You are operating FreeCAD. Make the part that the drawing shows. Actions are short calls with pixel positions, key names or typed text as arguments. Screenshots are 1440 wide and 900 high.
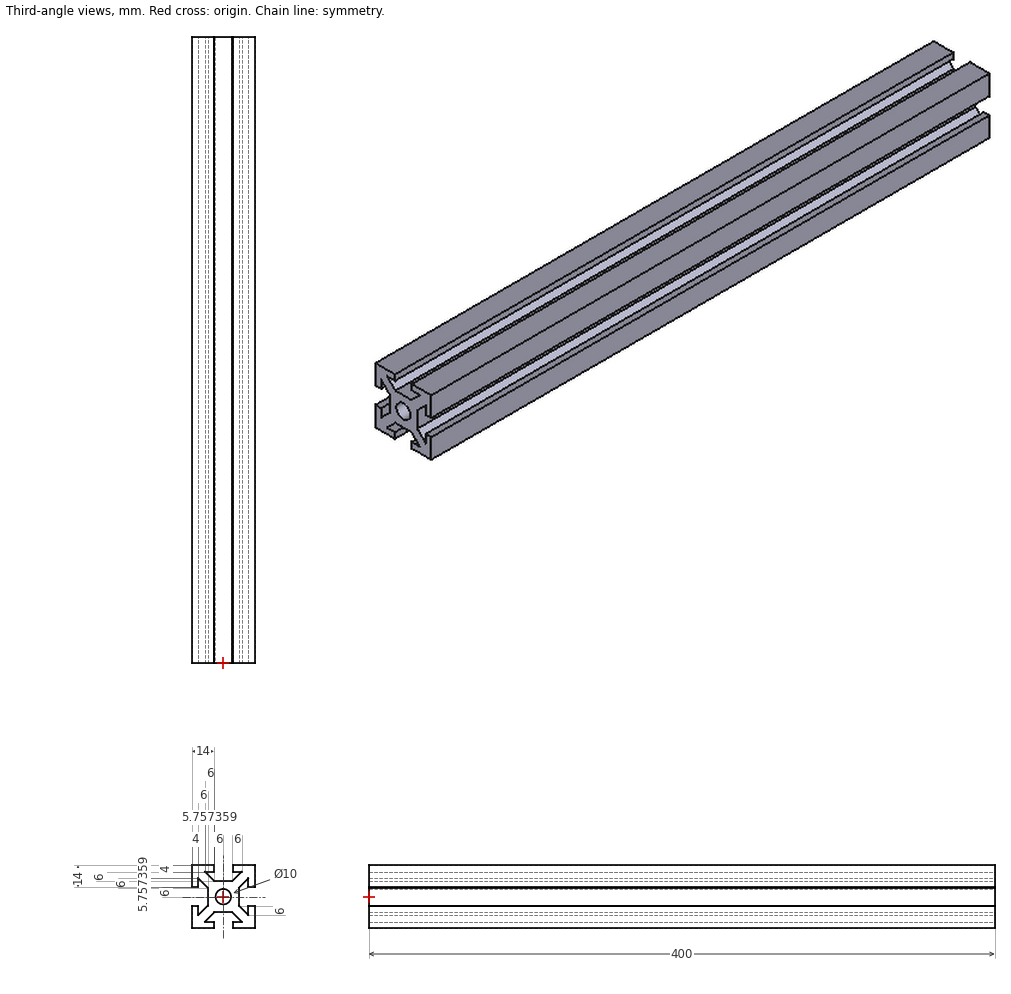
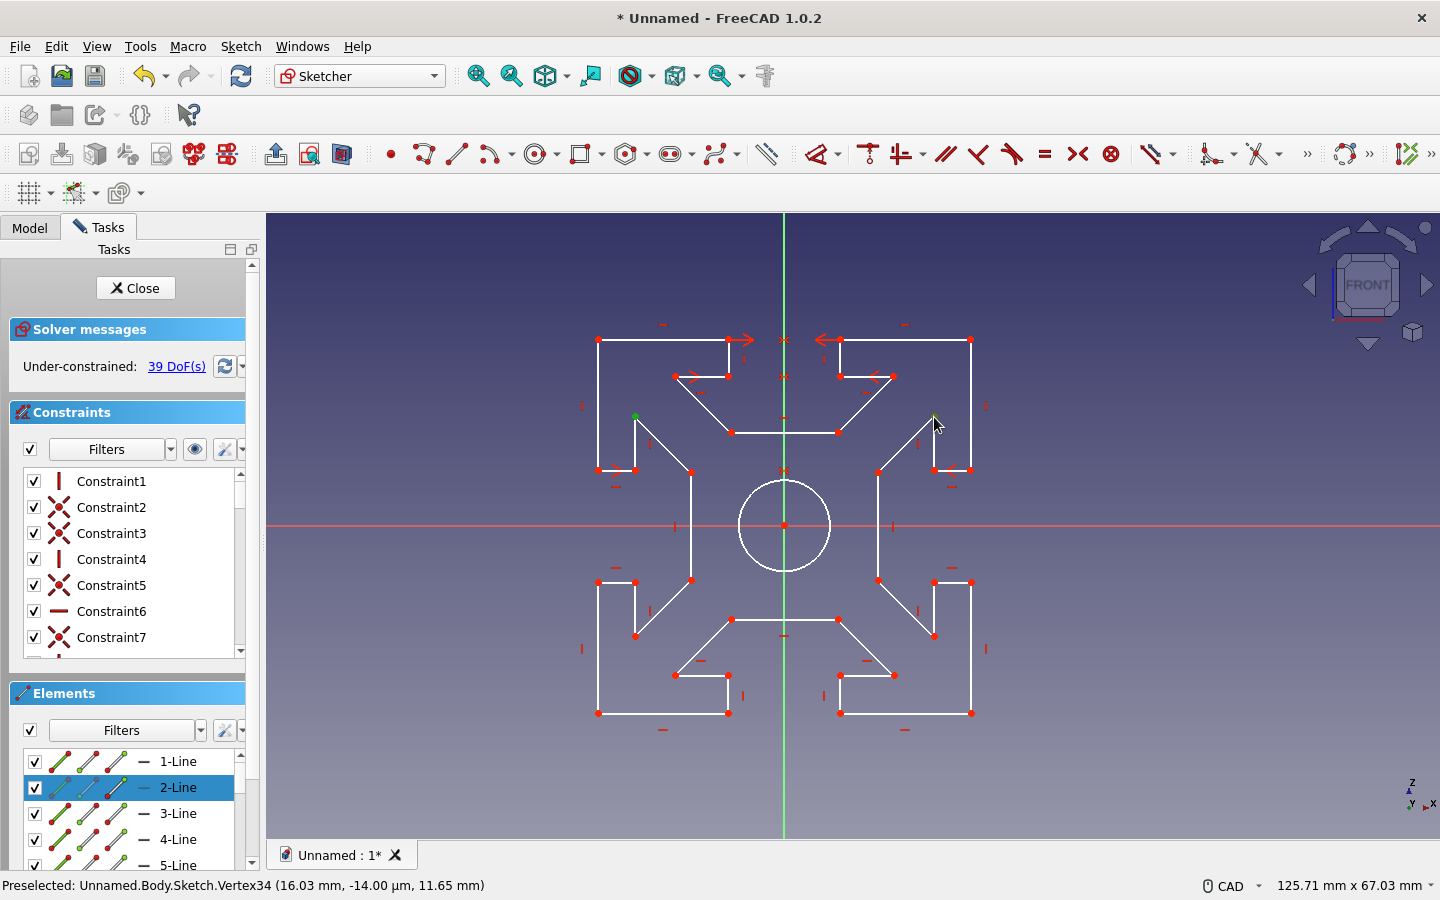
click(784, 770)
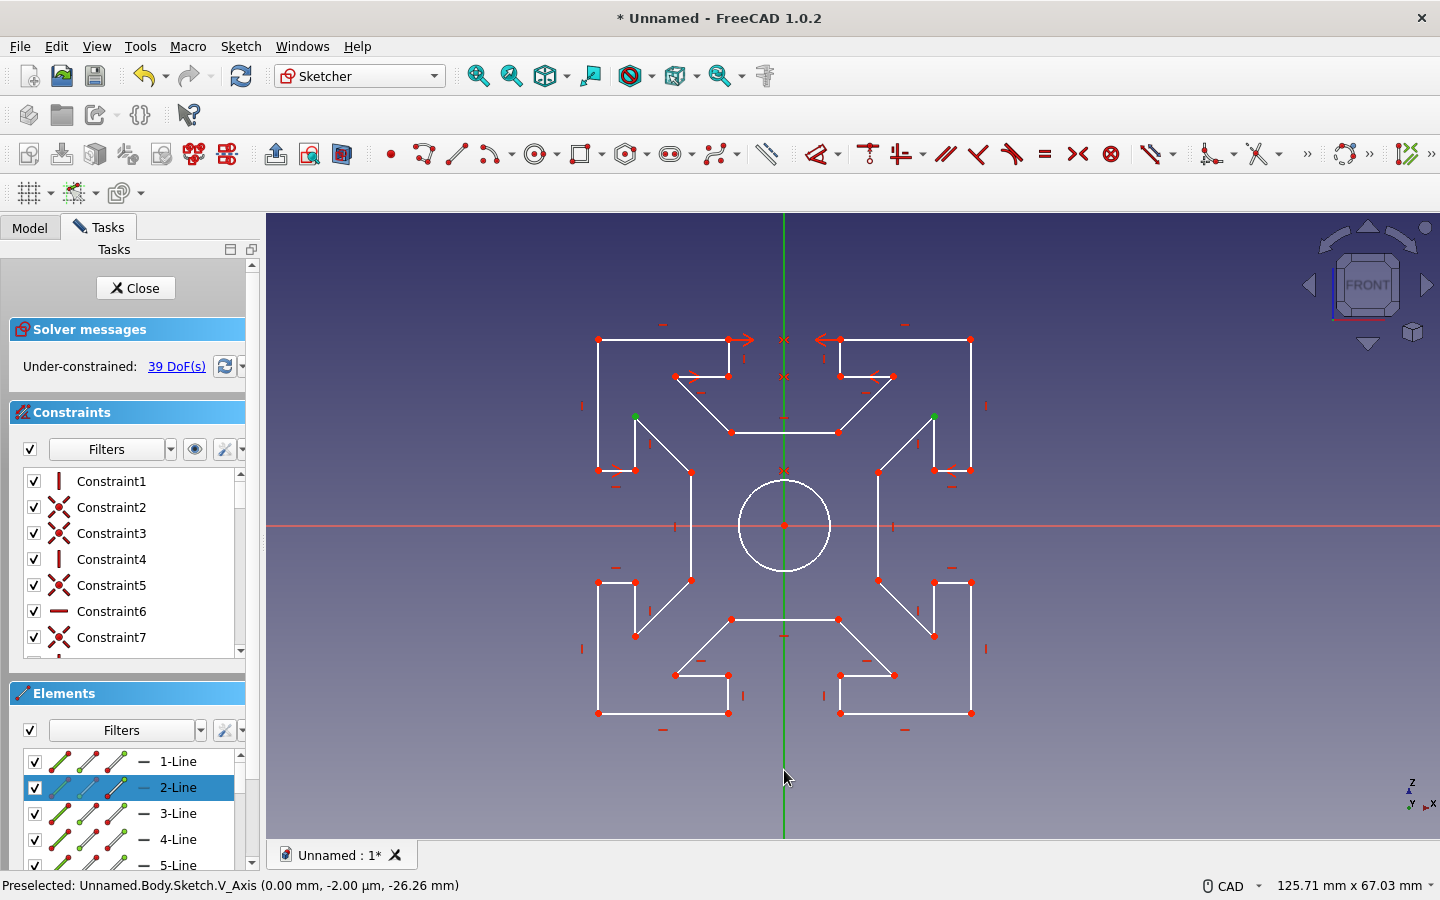
key(s)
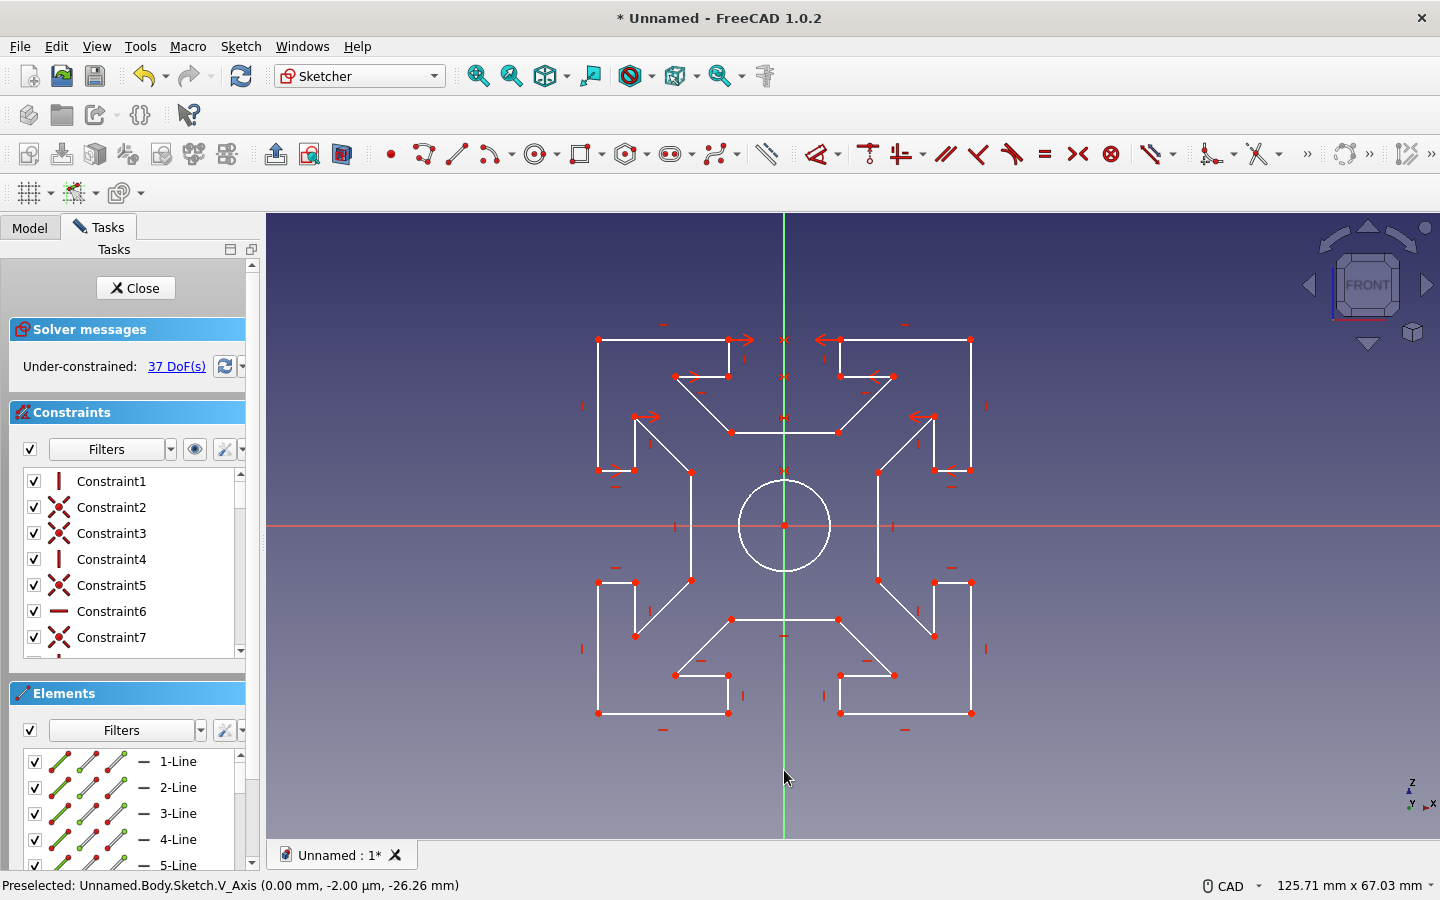
click(691, 473)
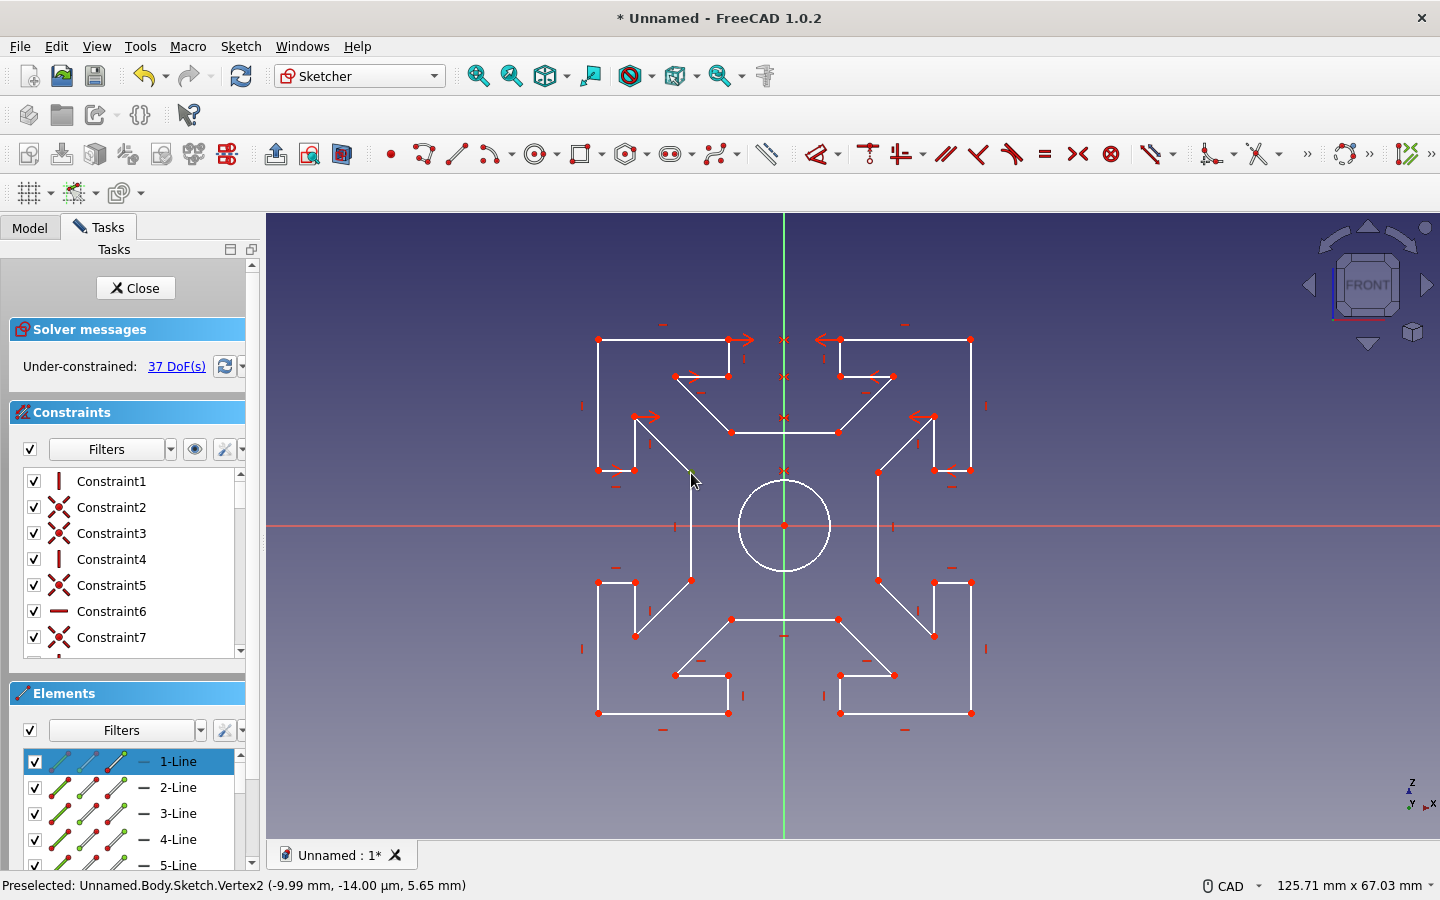
click(878, 473)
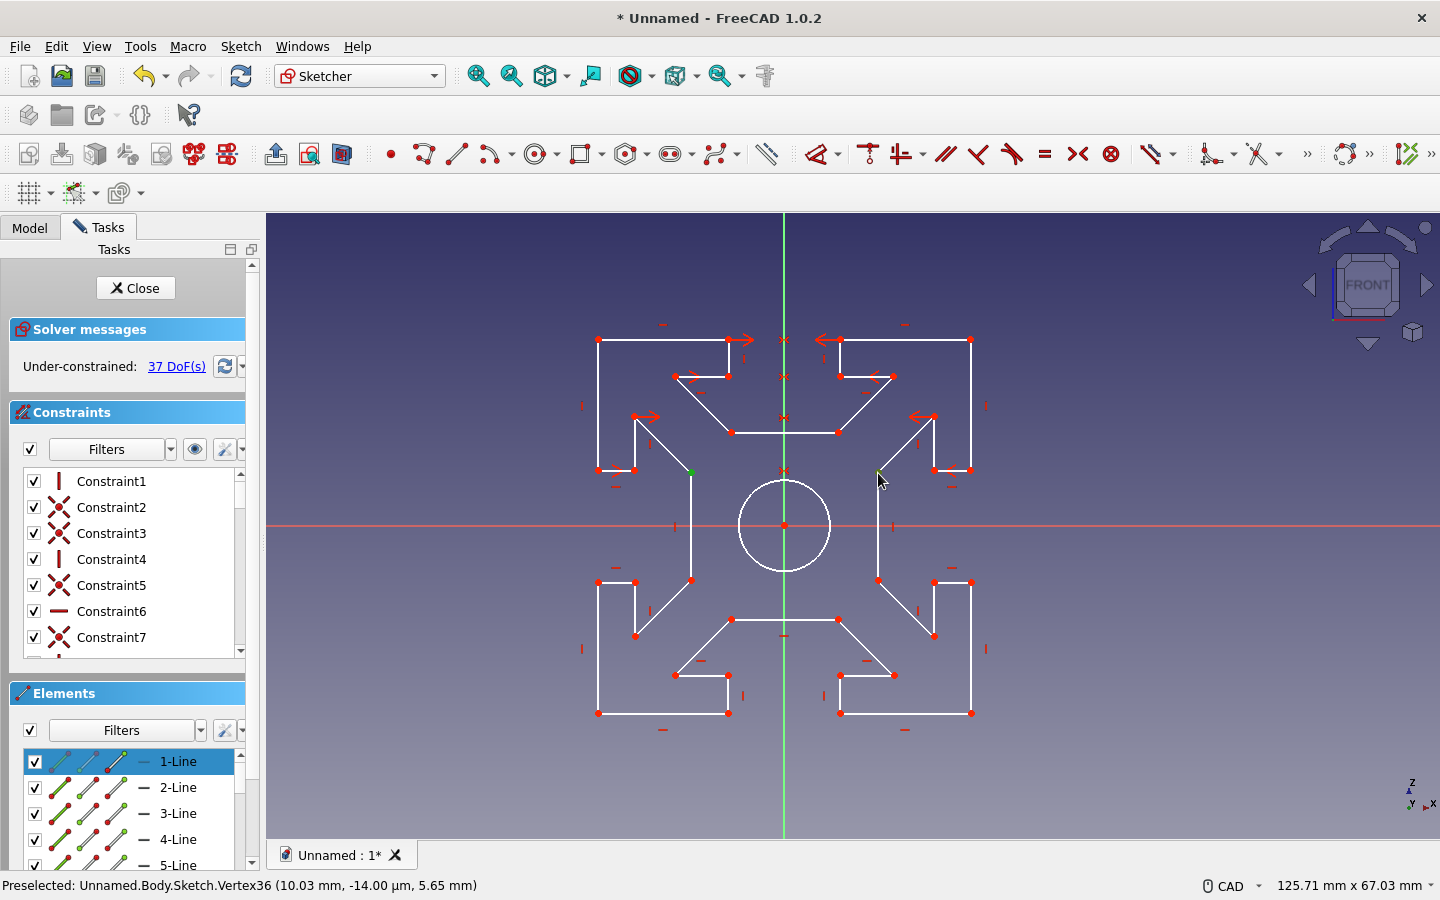
click(784, 770)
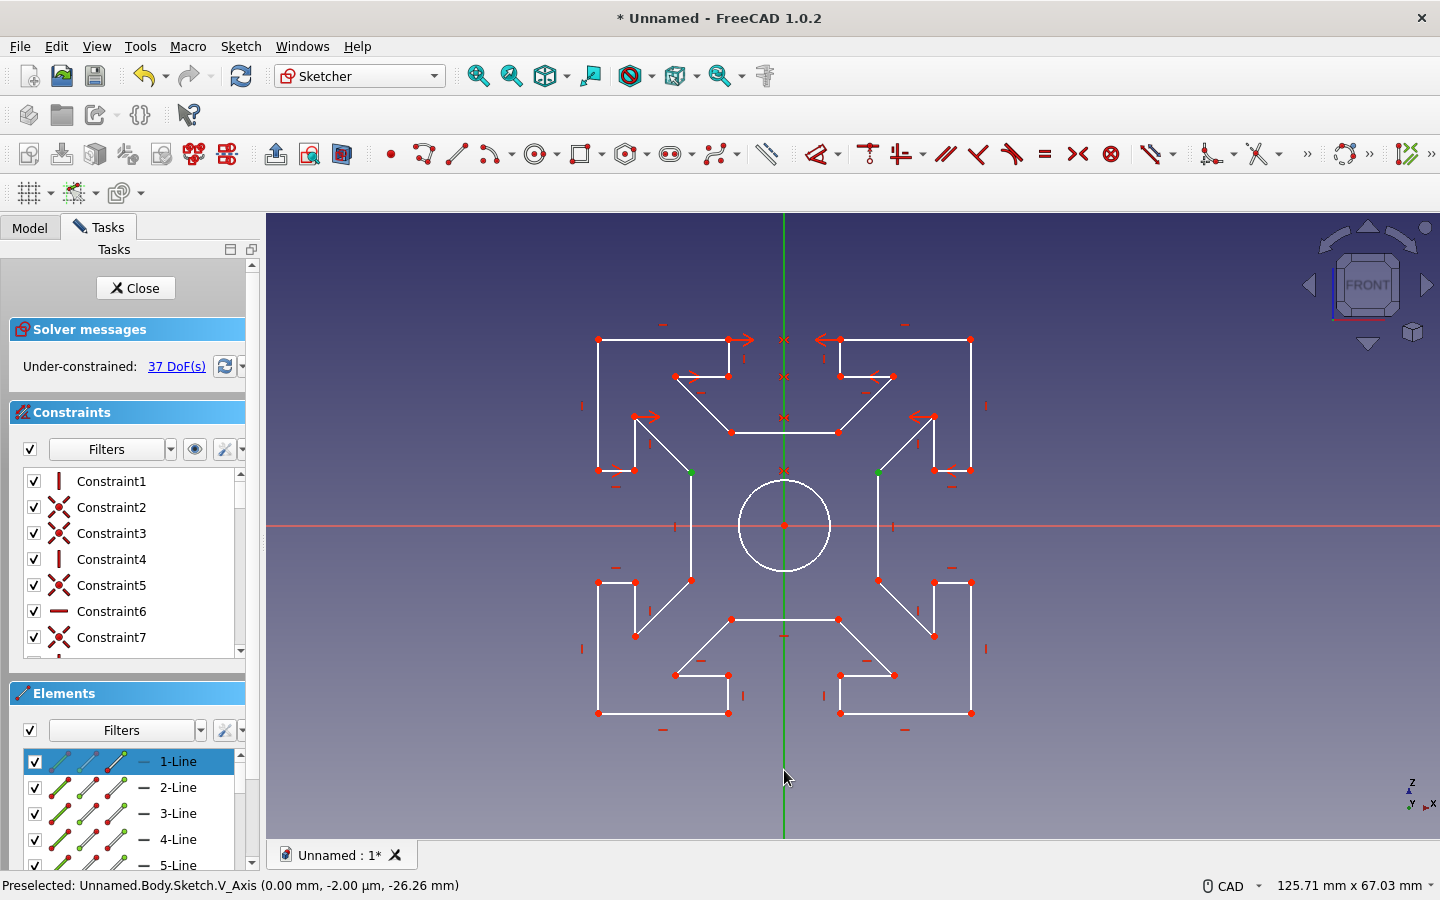
key(s)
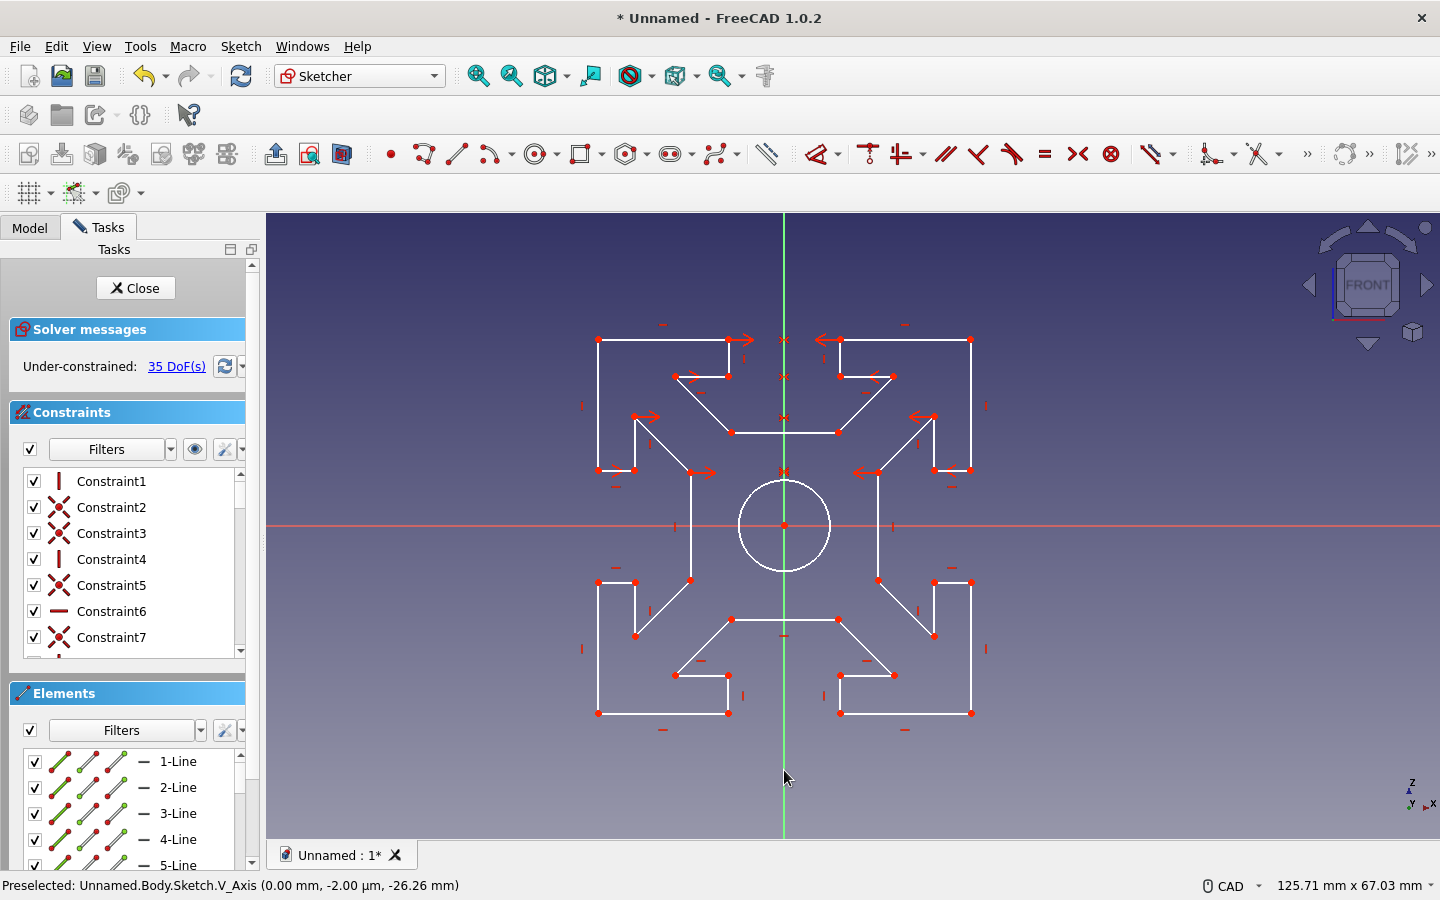
click(934, 417)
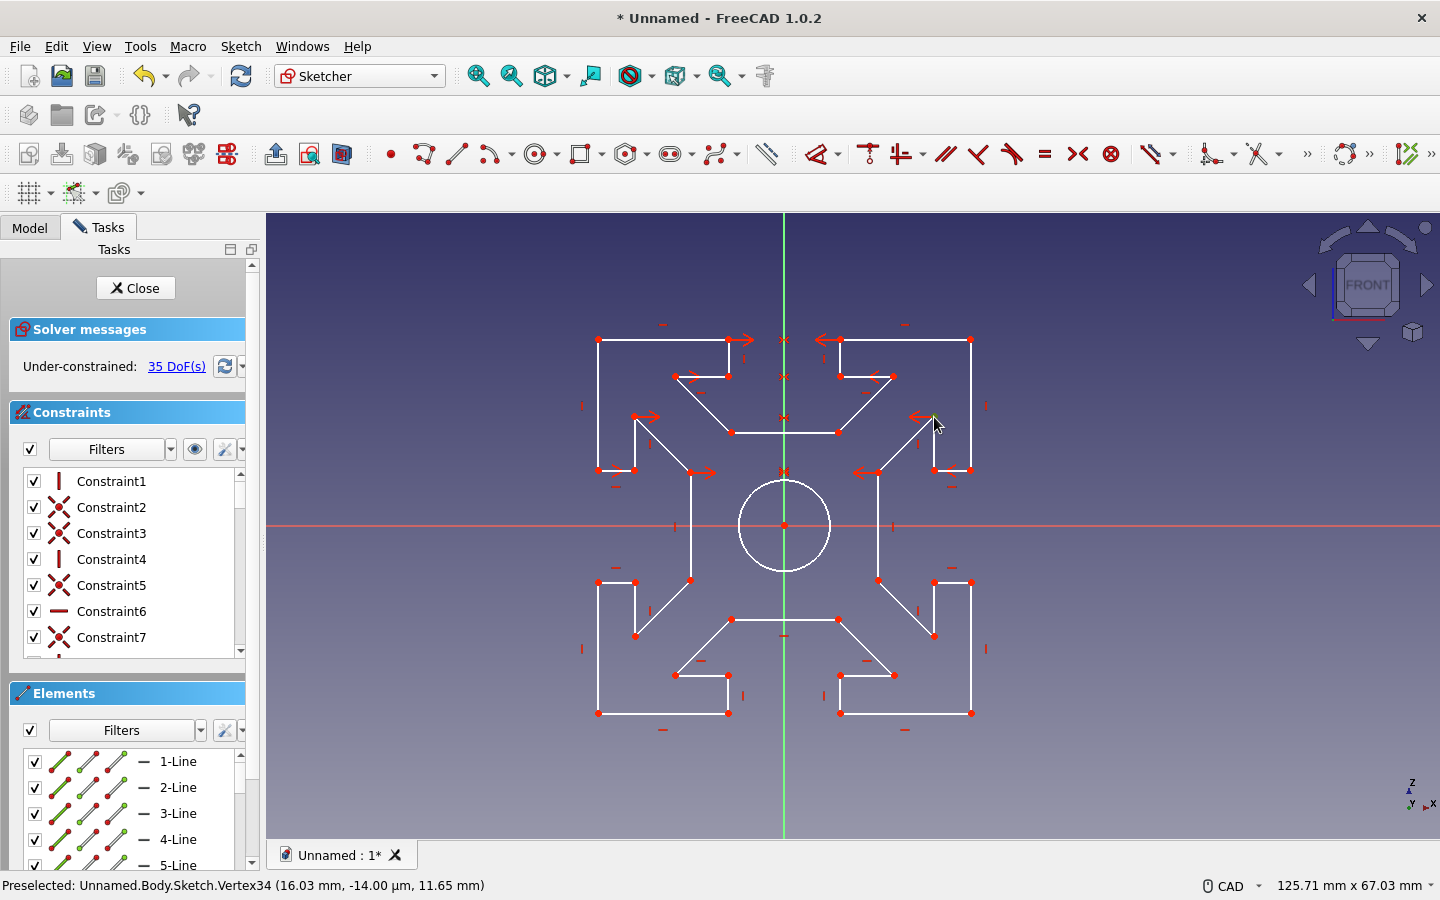
click(934, 637)